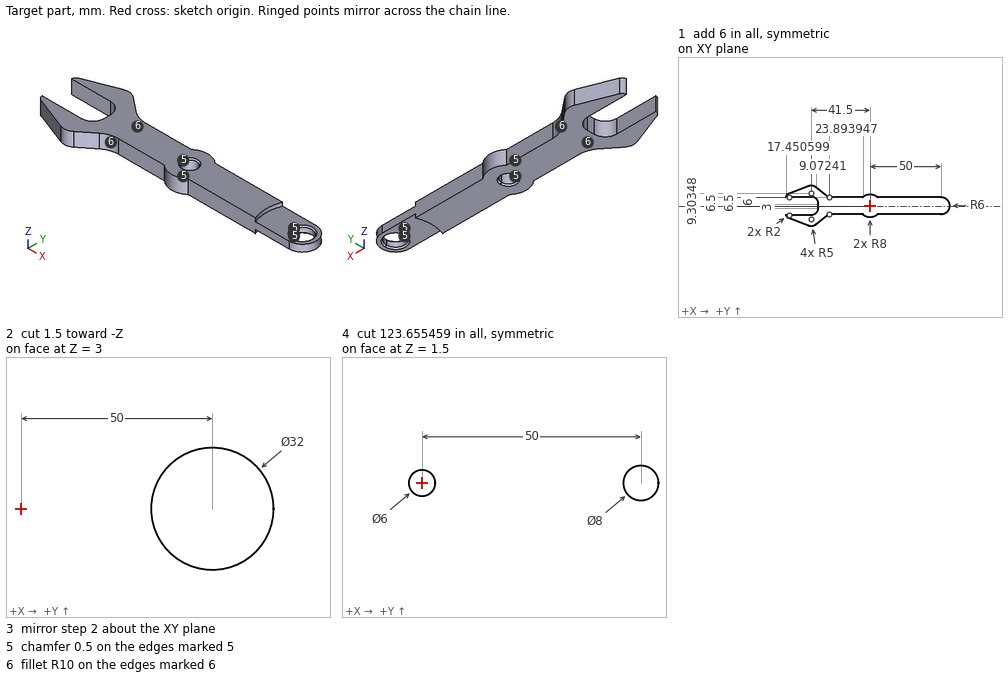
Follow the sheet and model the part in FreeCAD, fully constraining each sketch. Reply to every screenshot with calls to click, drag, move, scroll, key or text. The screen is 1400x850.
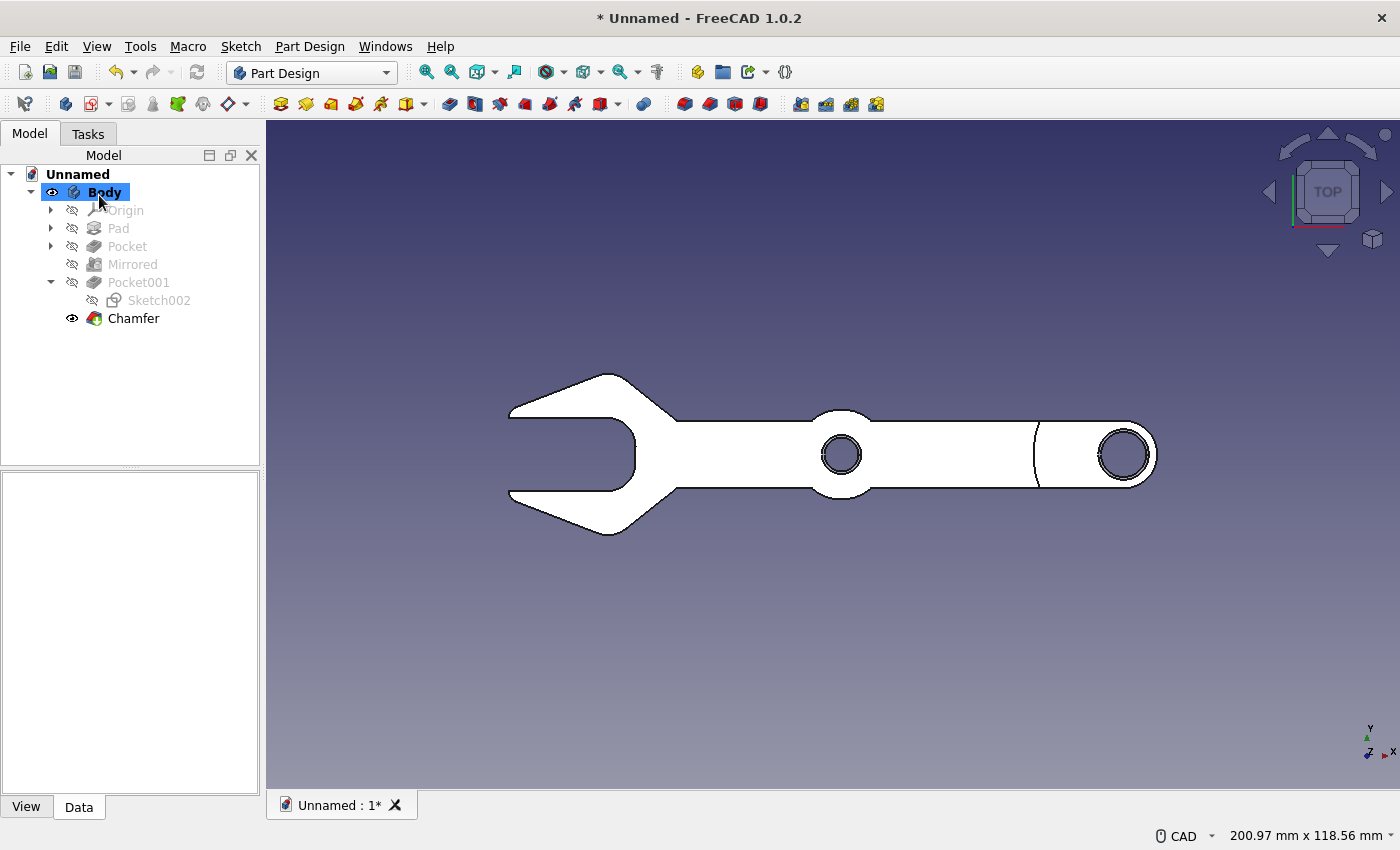
key(1)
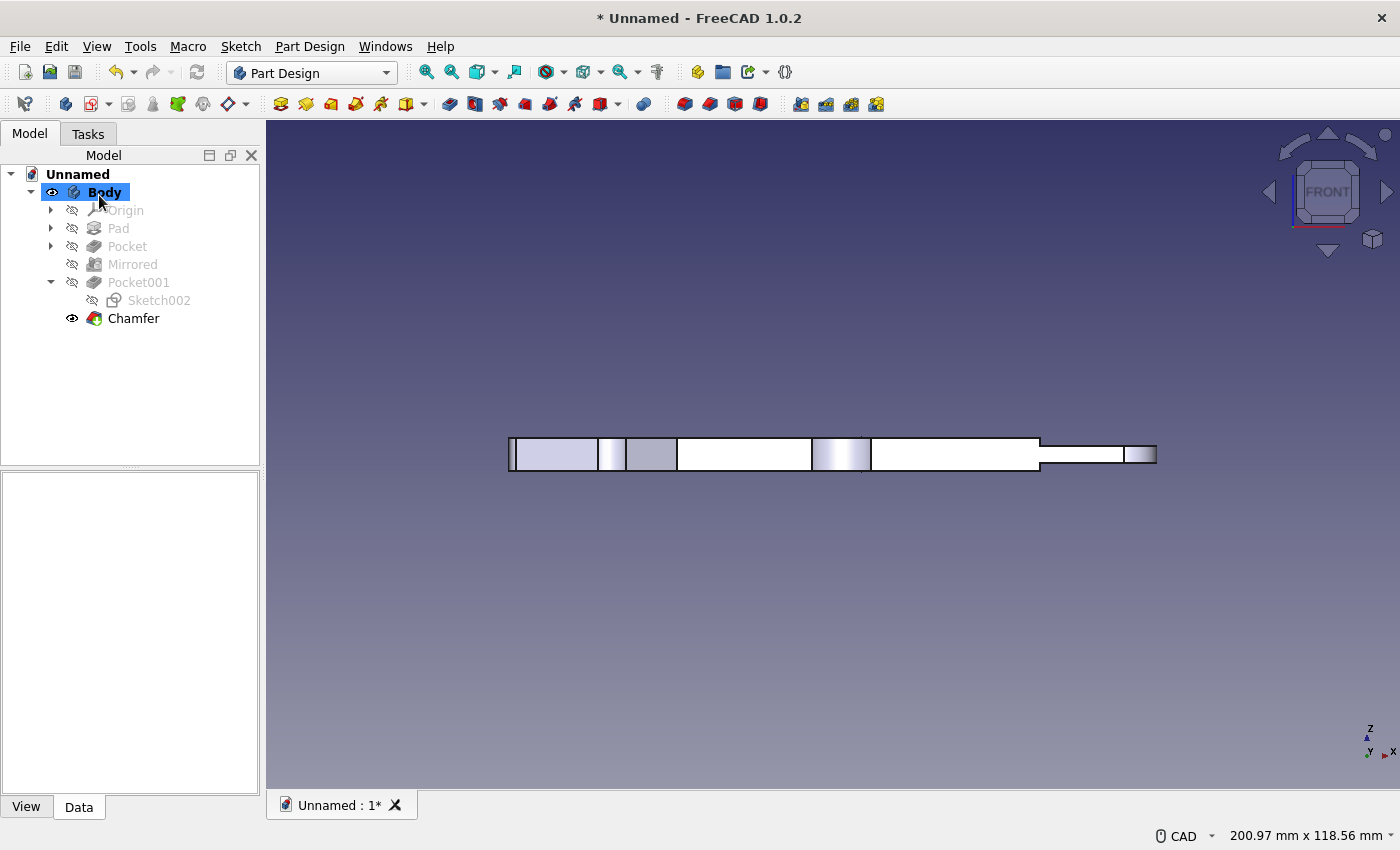
key(3)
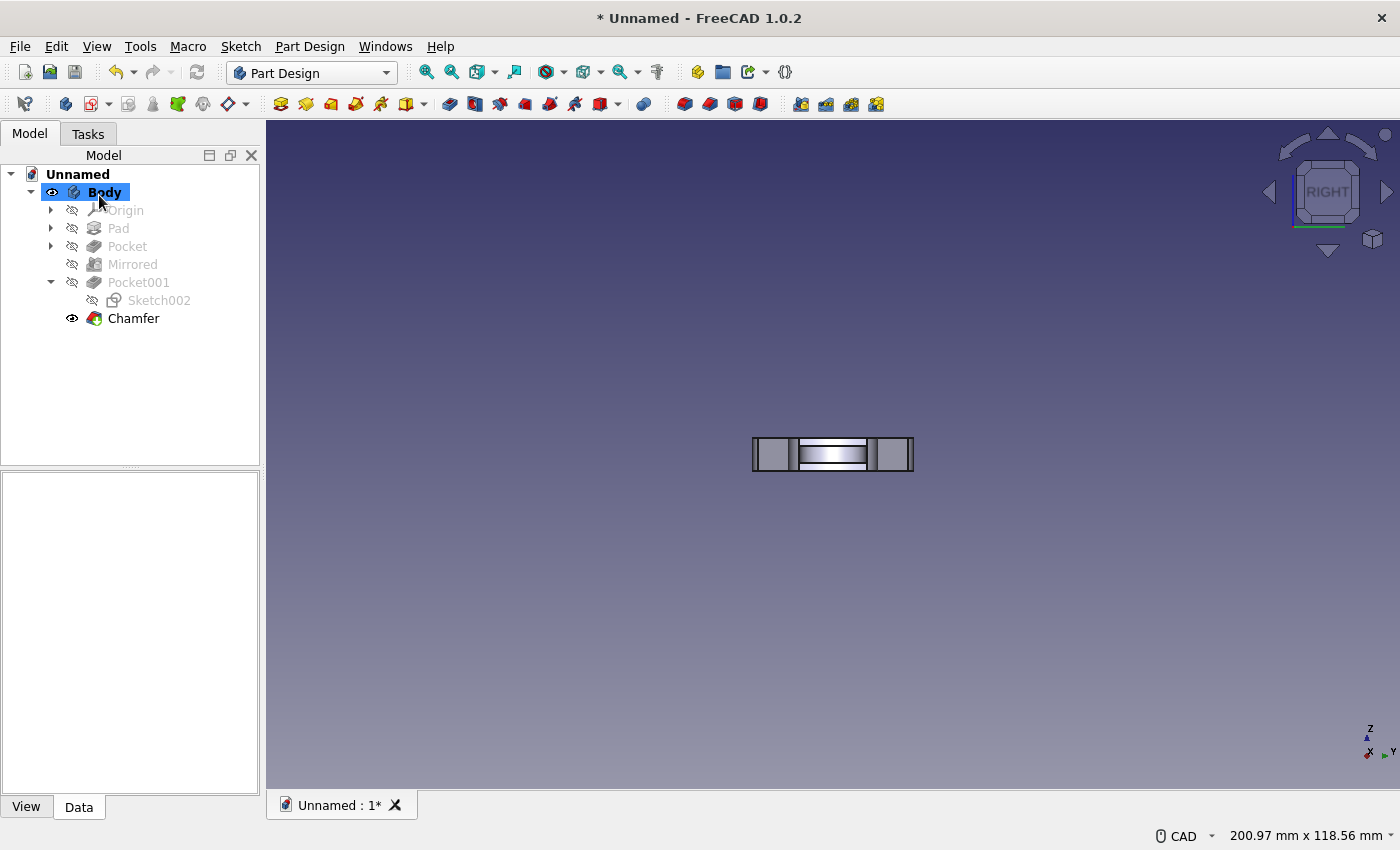
click(427, 72)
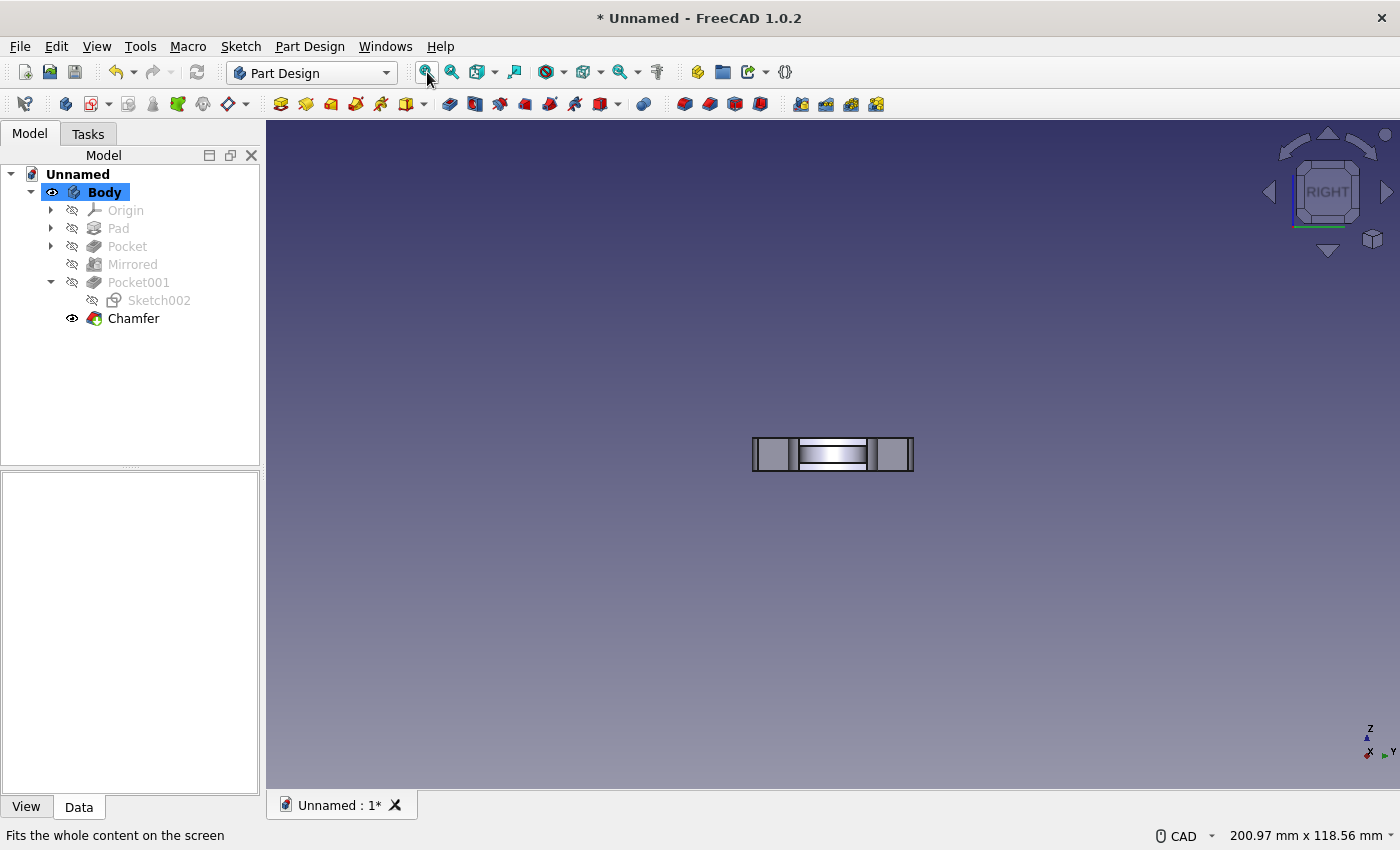
key(5)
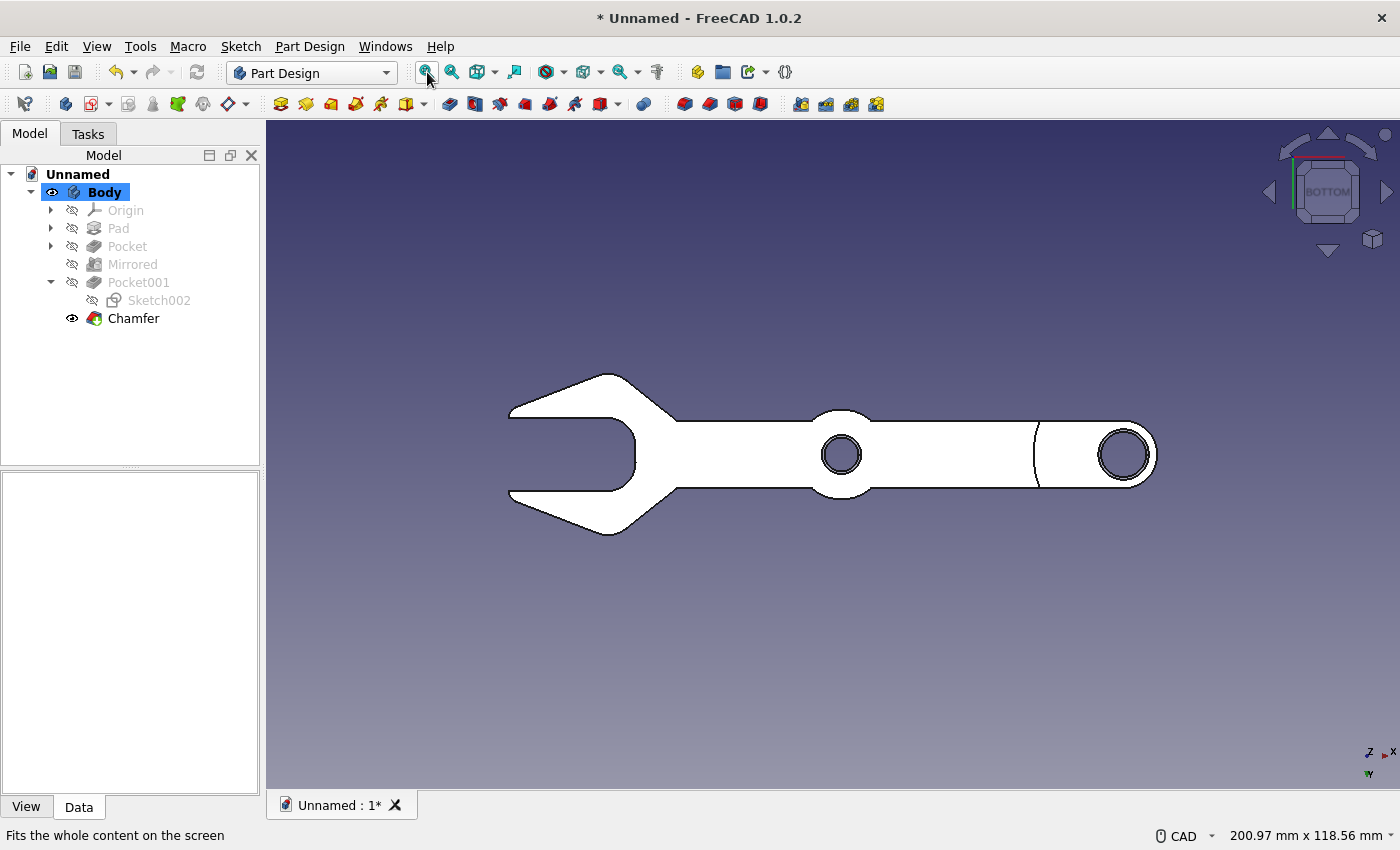
key(4)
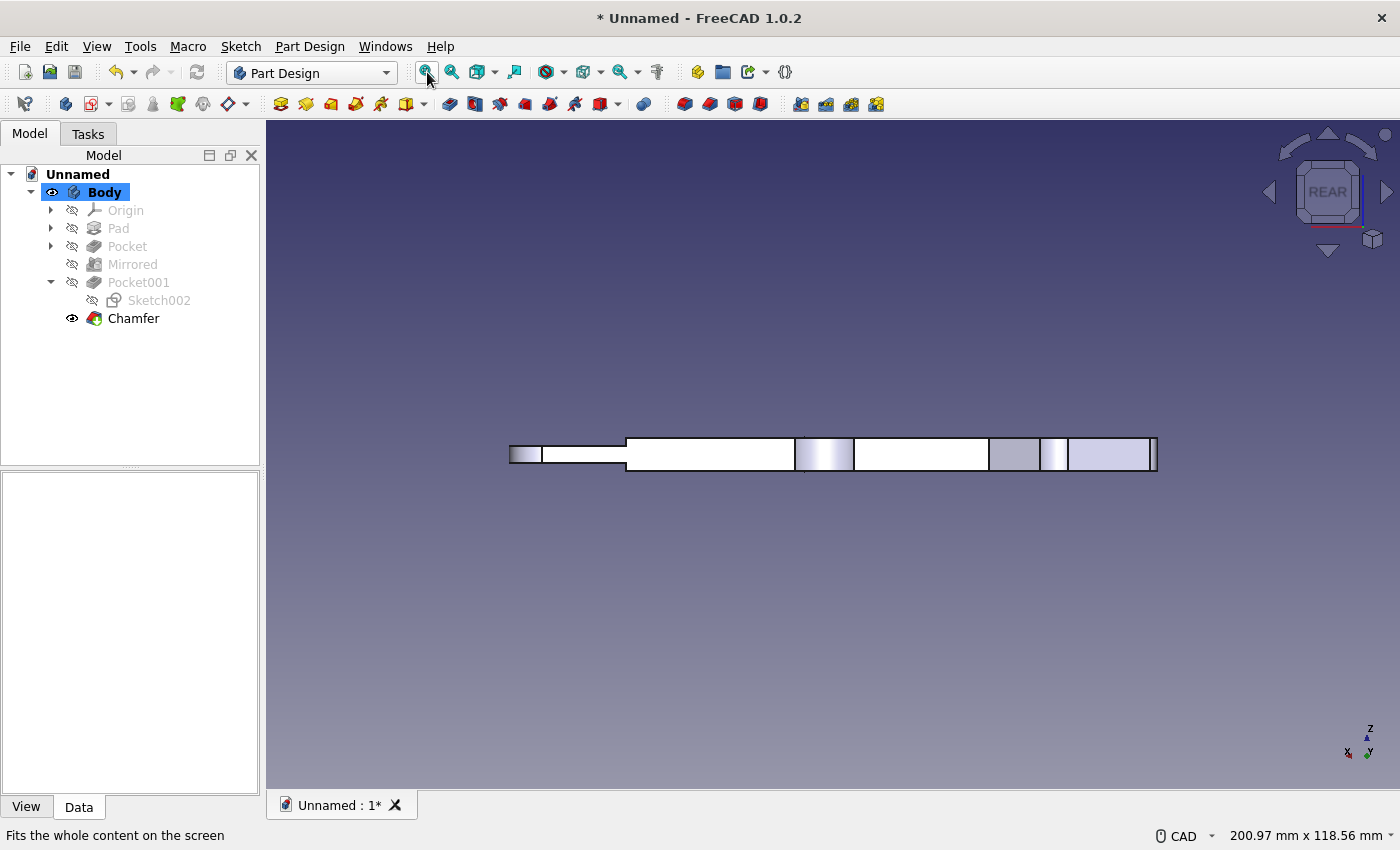
key(6)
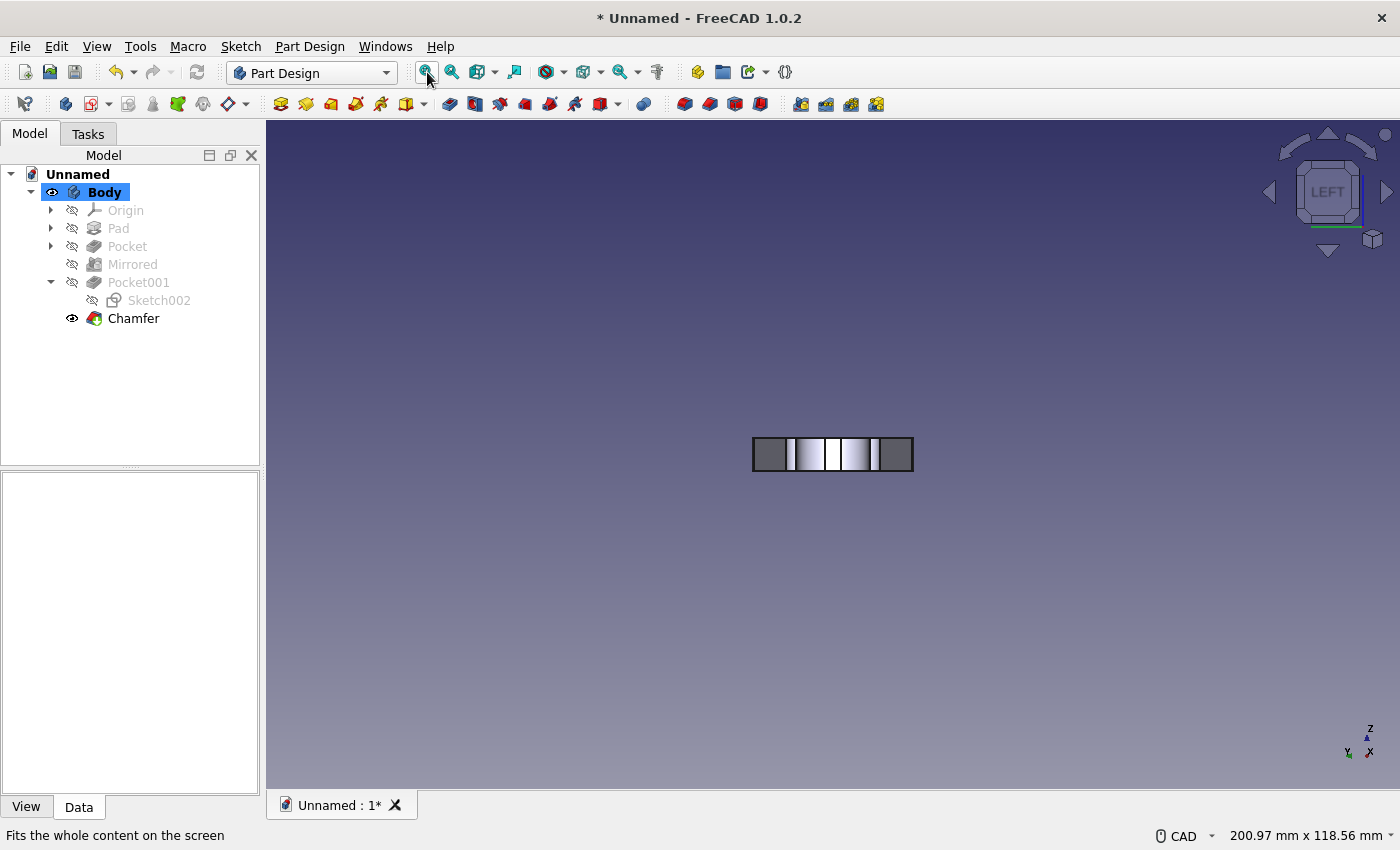
click(427, 72)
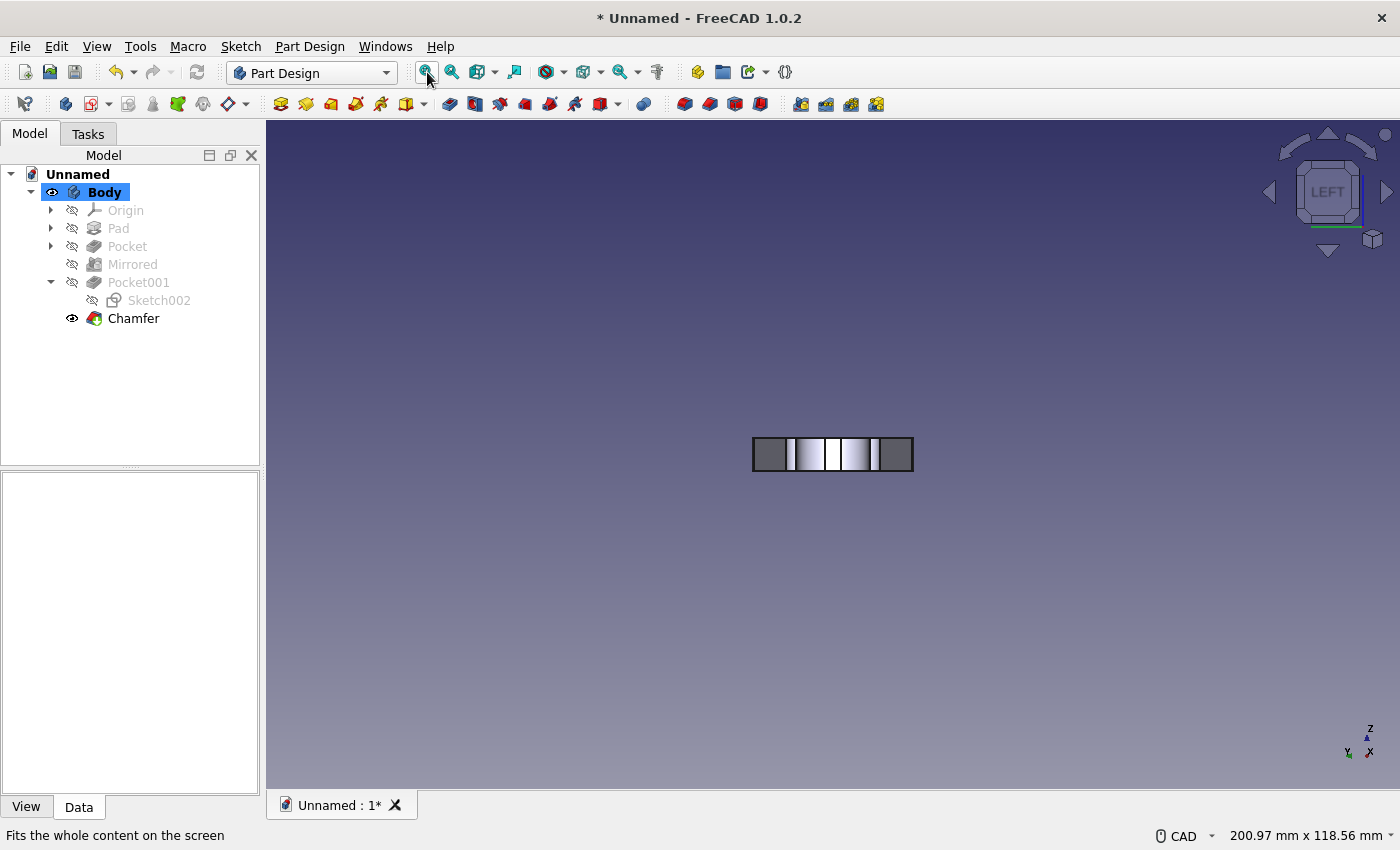
key(v)
key(3)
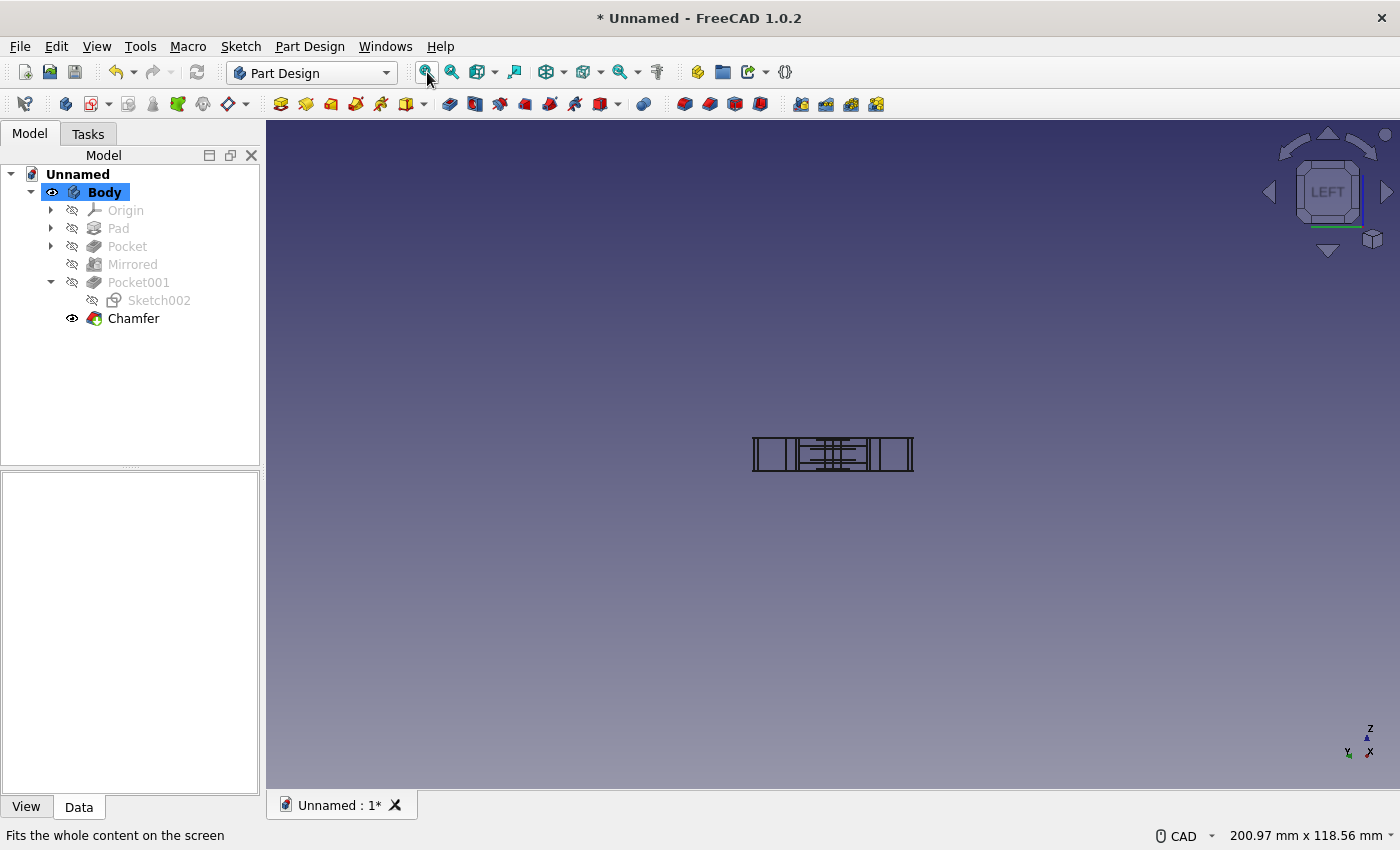
key(0)